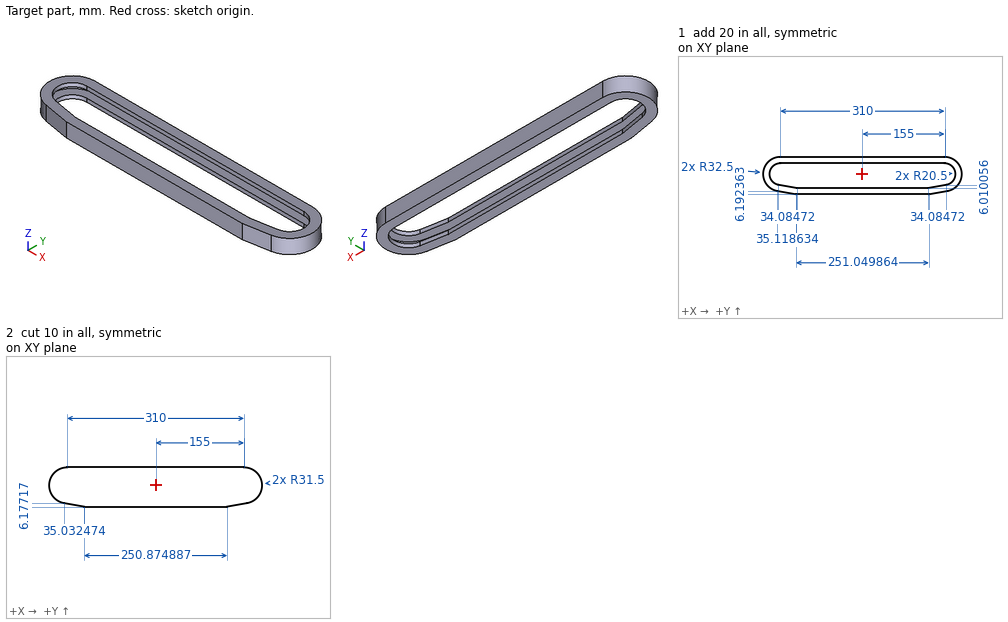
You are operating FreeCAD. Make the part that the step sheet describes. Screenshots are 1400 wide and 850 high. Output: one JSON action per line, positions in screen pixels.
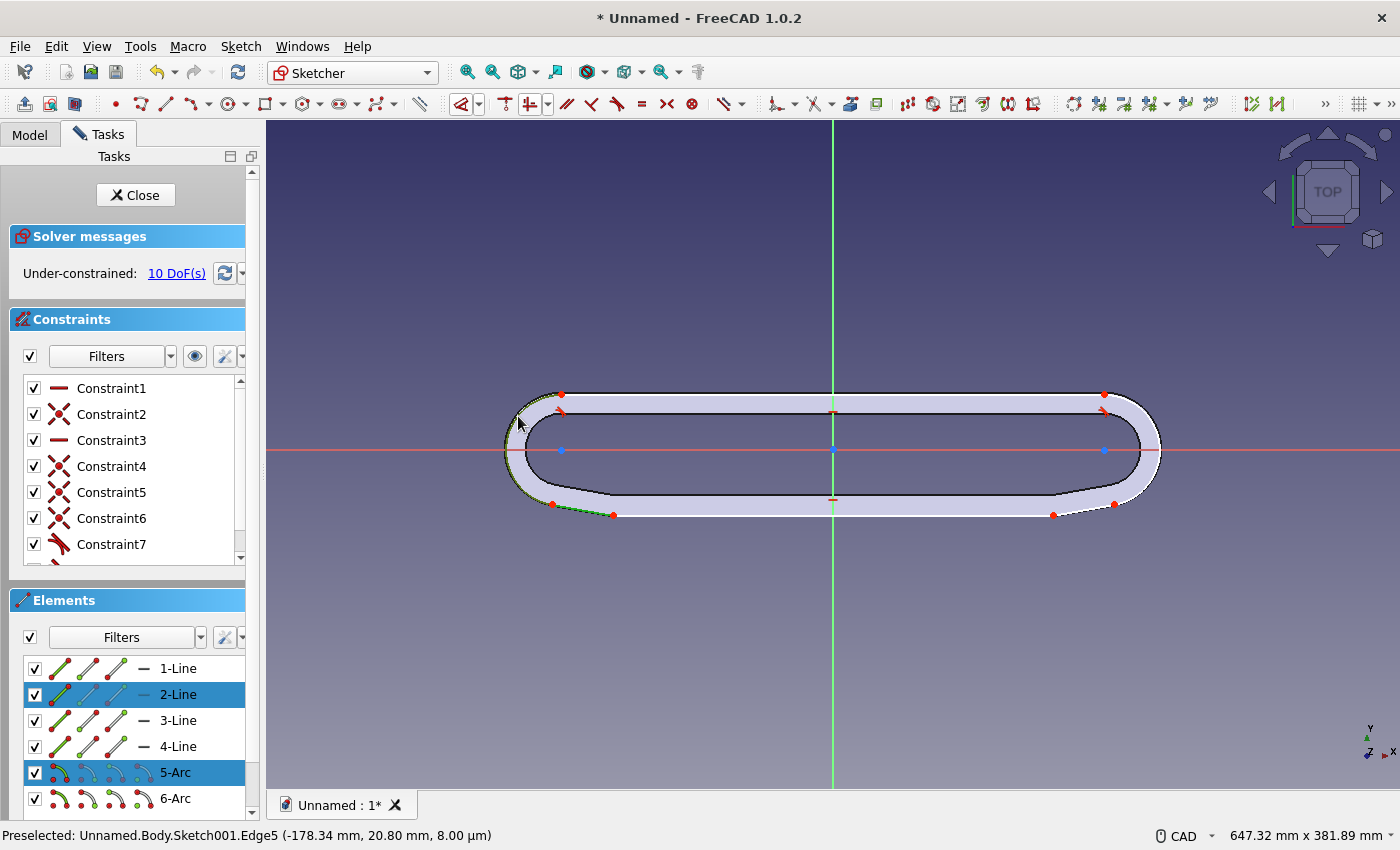
{"action": "left_click", "coordinate": [617, 104]}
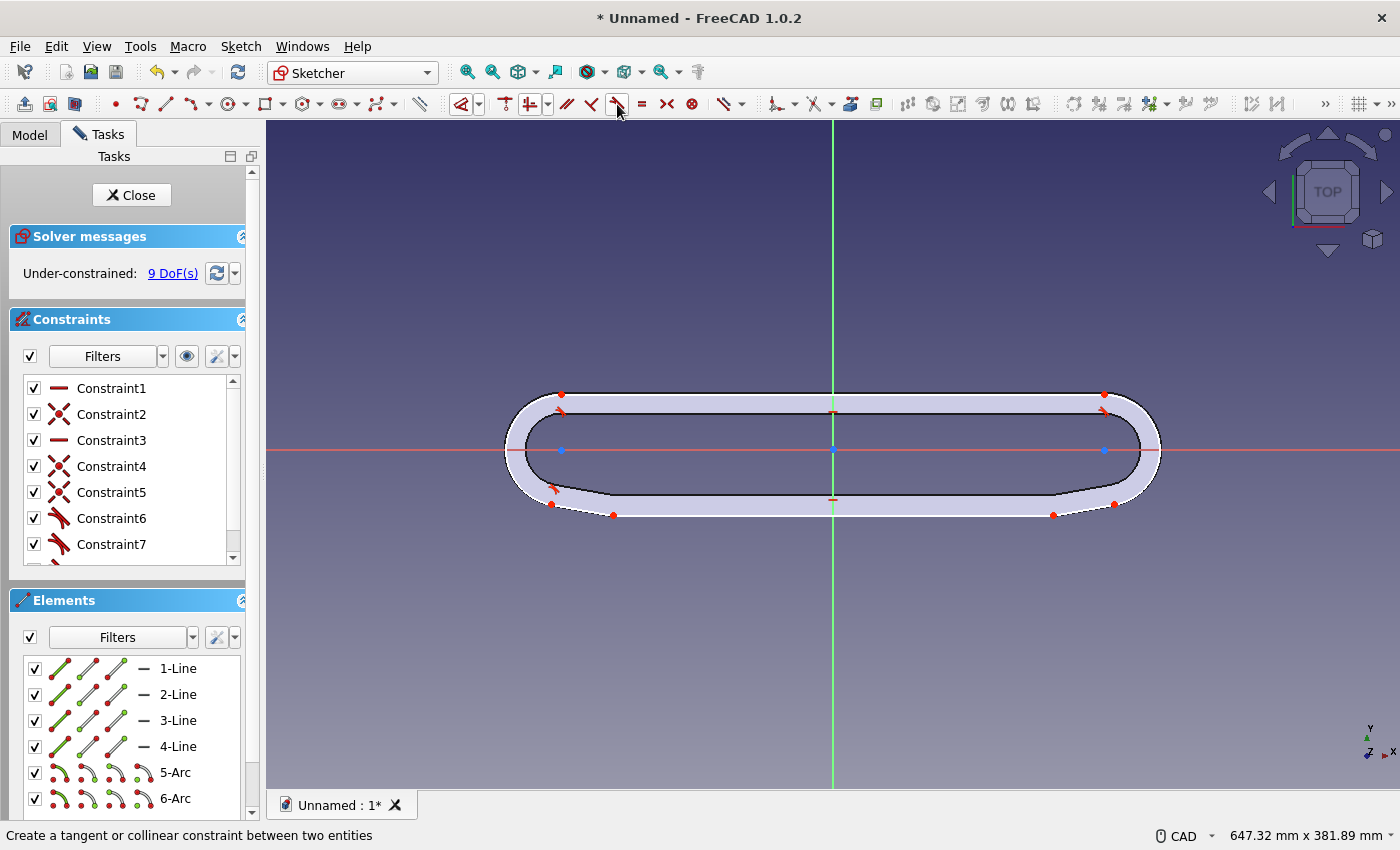
{"action": "left_click", "coordinate": [1071, 513]}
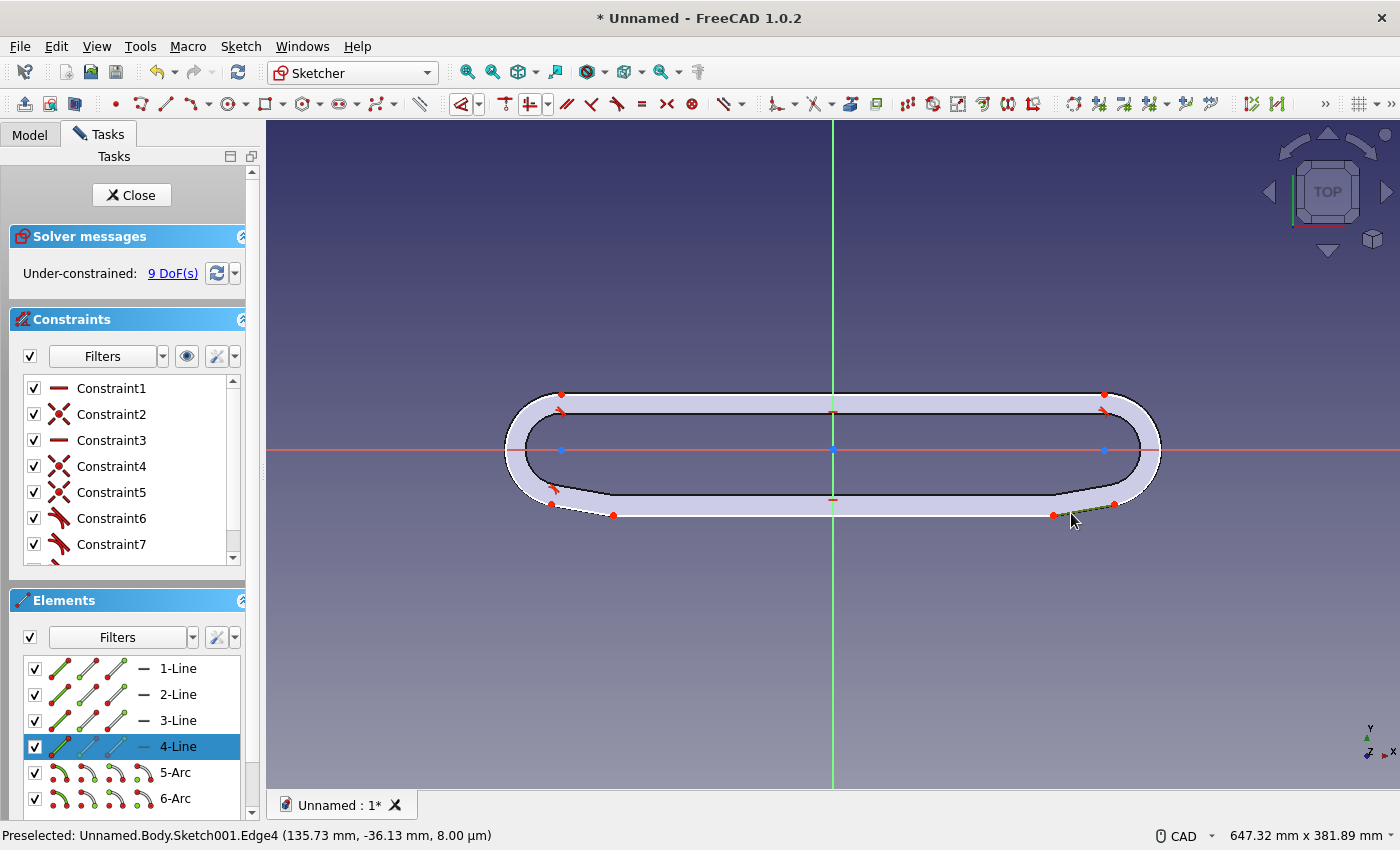
{"action": "left_click", "coordinate": [1153, 477]}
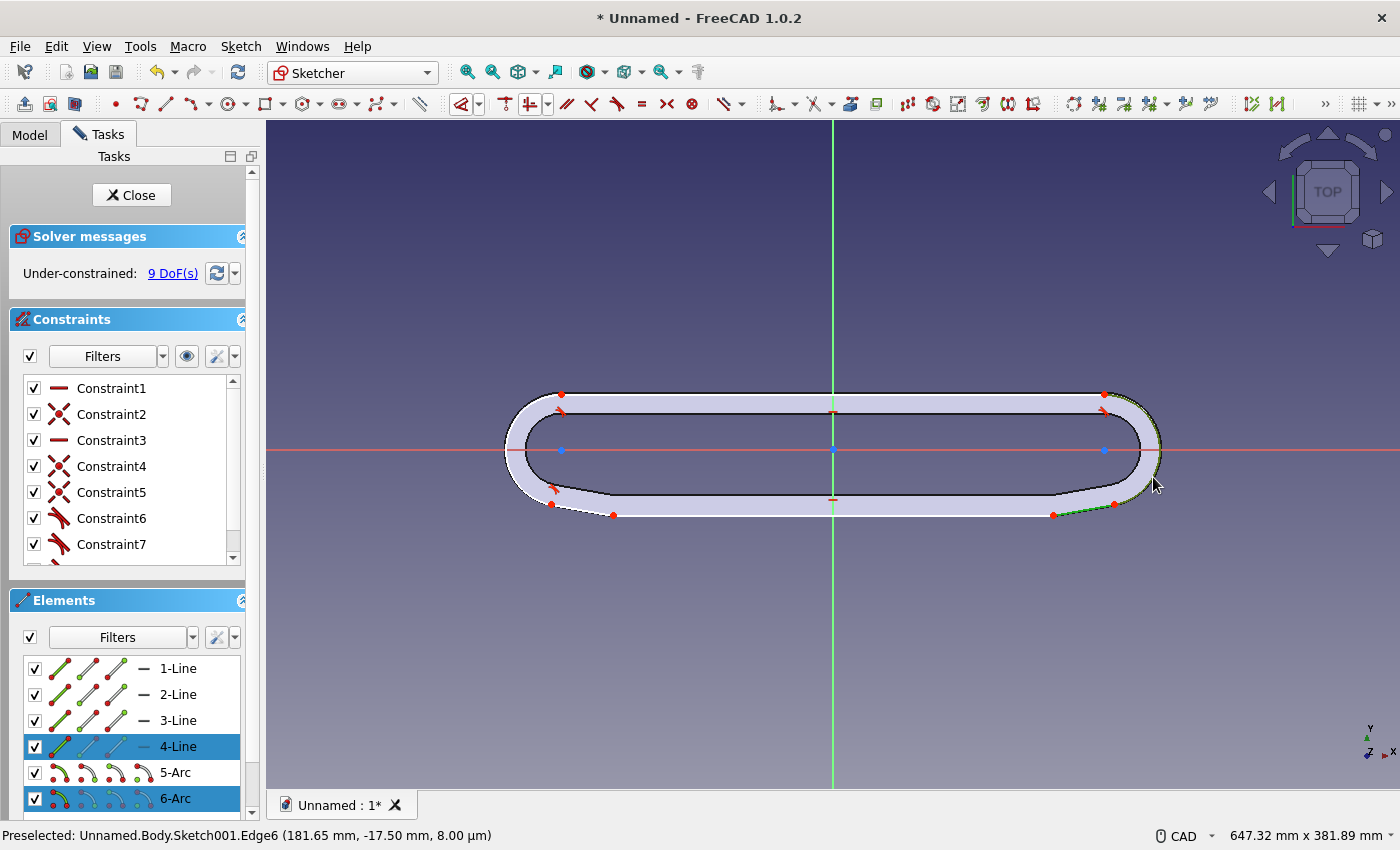
{"action": "key", "text": "t"}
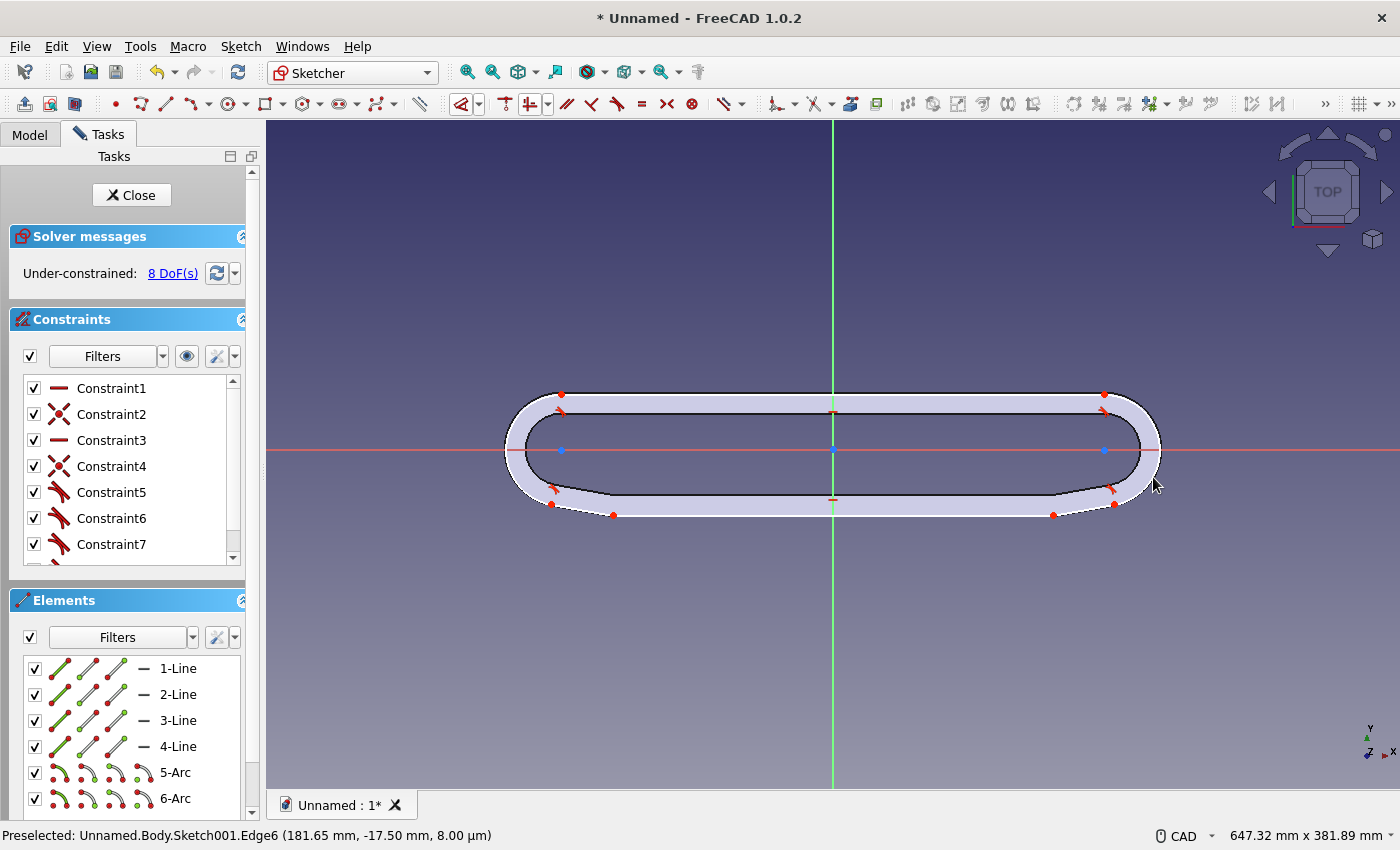
{"action": "left_click", "coordinate": [518, 416]}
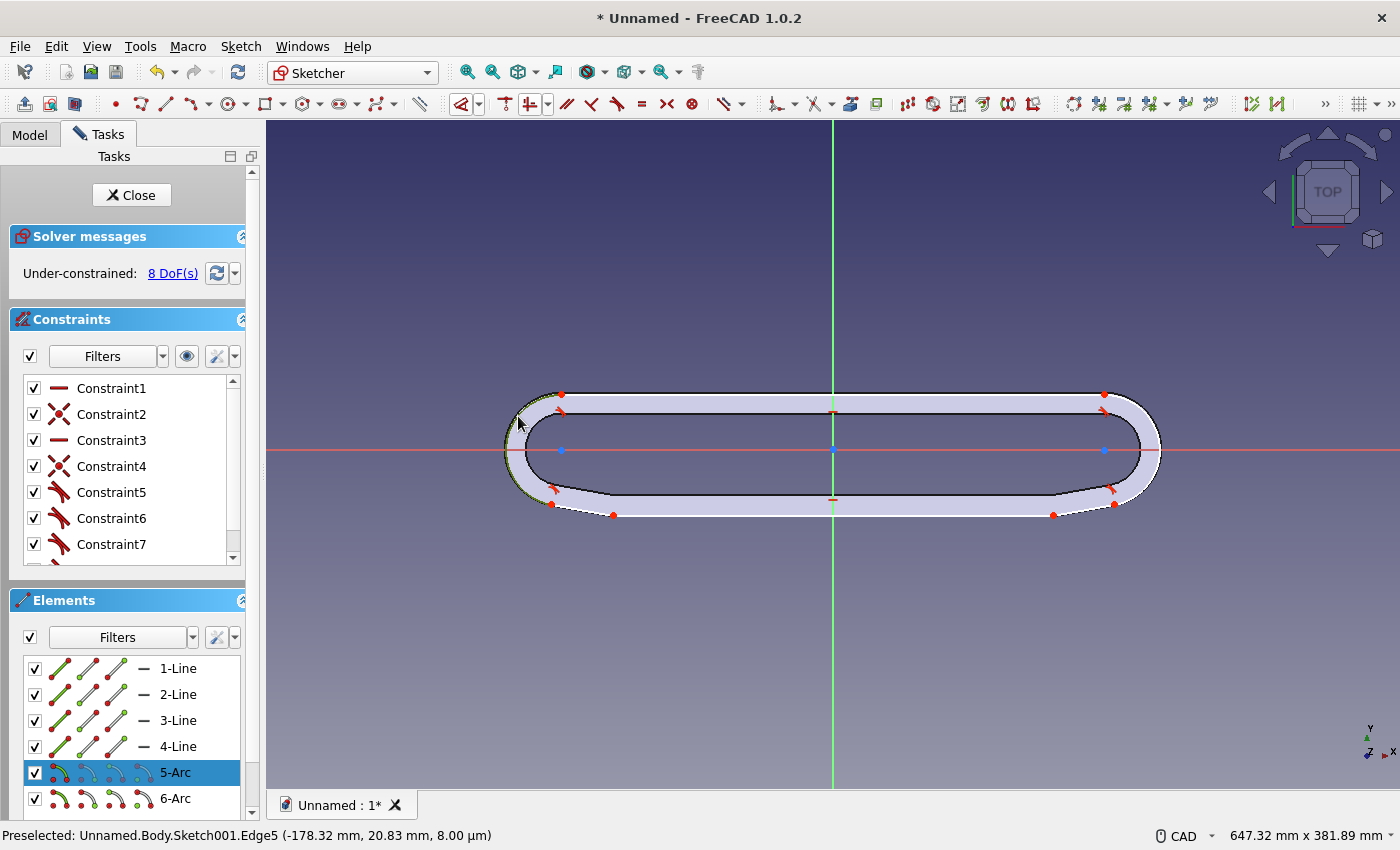
{"action": "left_click", "coordinate": [1153, 477]}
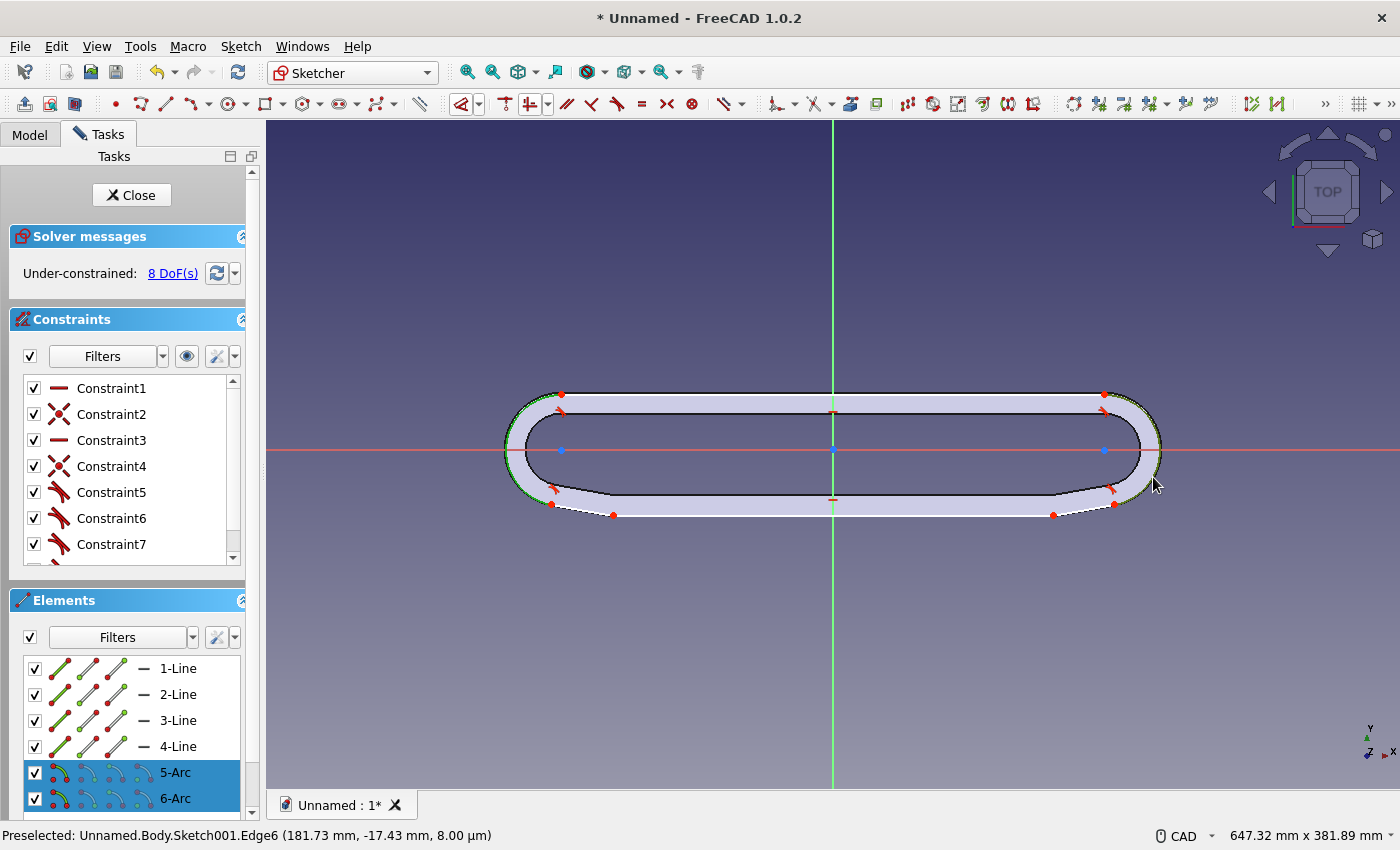
{"action": "left_click", "coordinate": [642, 104]}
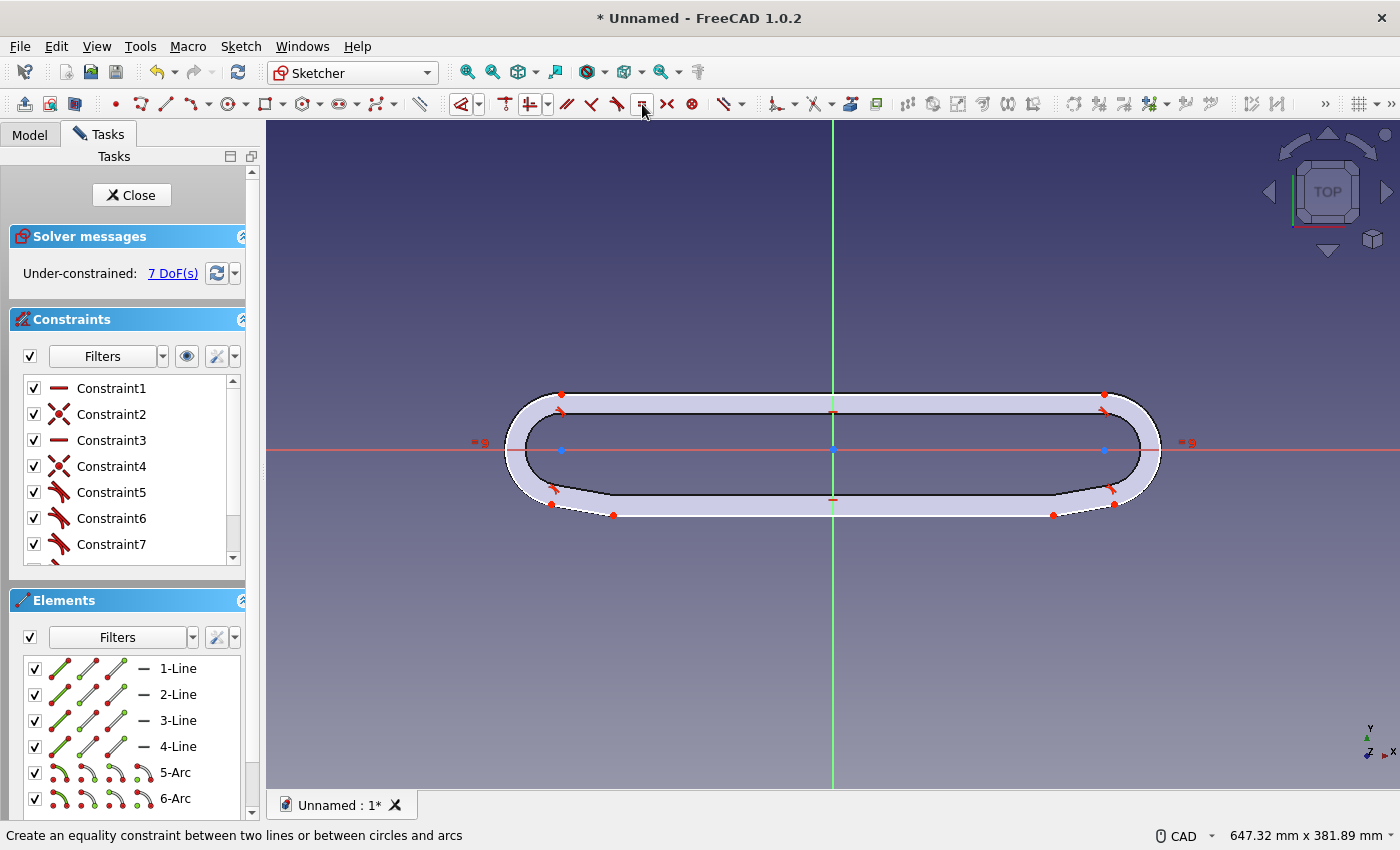
{"action": "left_click", "coordinate": [562, 450]}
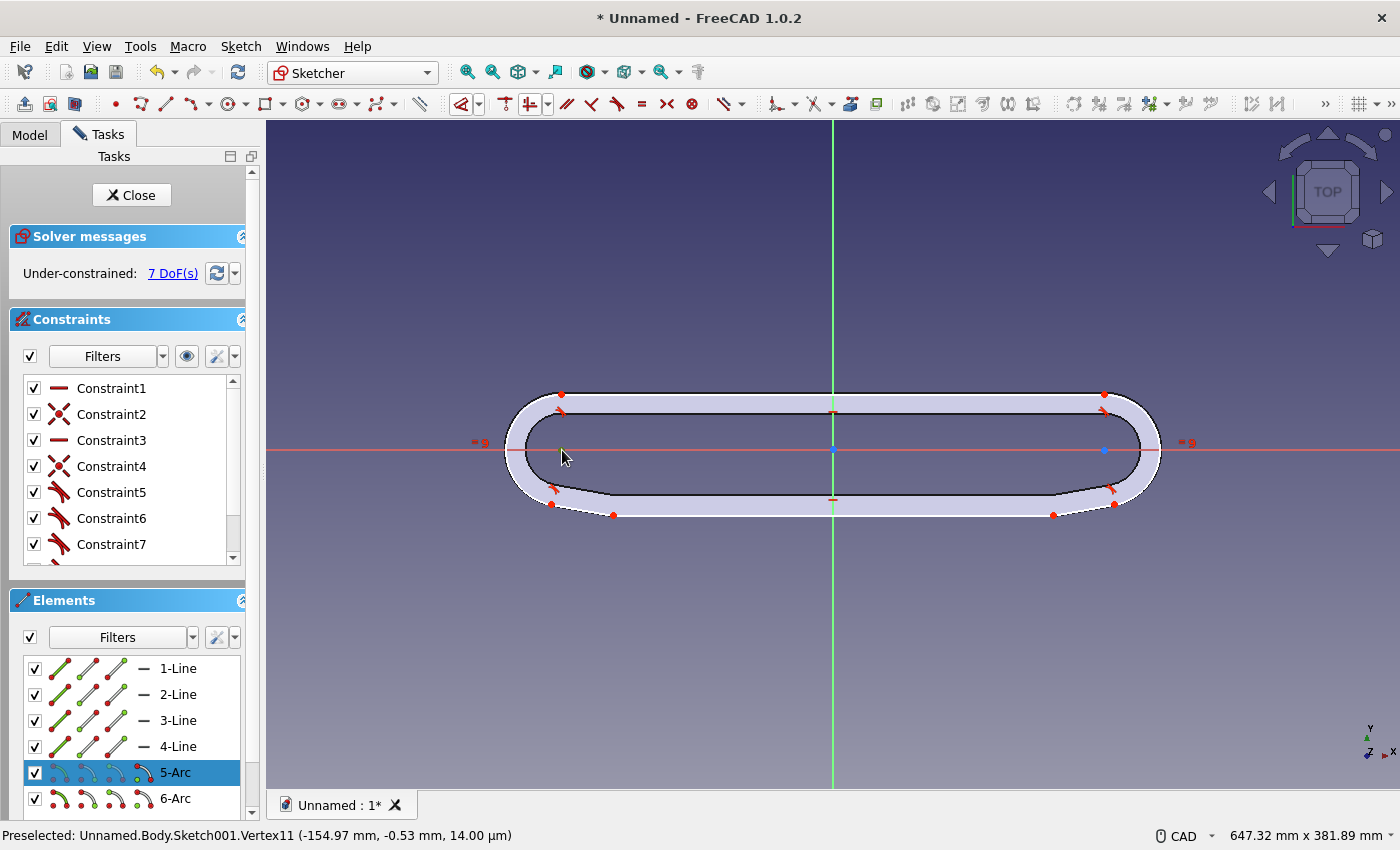
{"action": "left_click", "coordinate": [361, 450]}